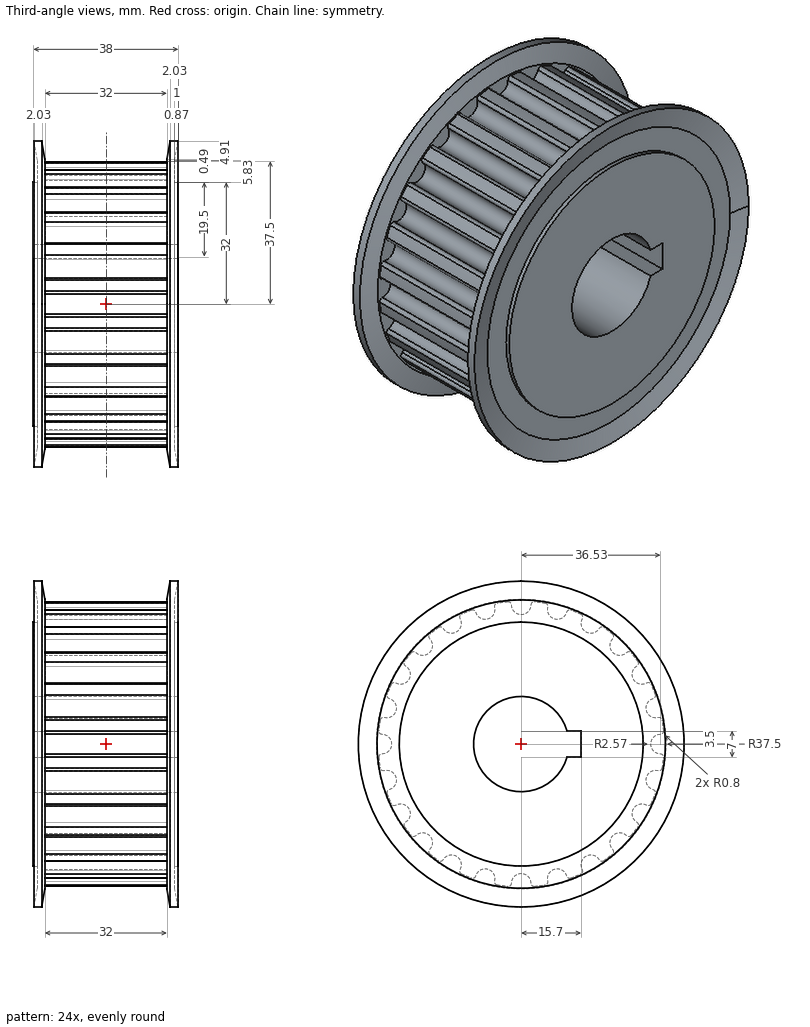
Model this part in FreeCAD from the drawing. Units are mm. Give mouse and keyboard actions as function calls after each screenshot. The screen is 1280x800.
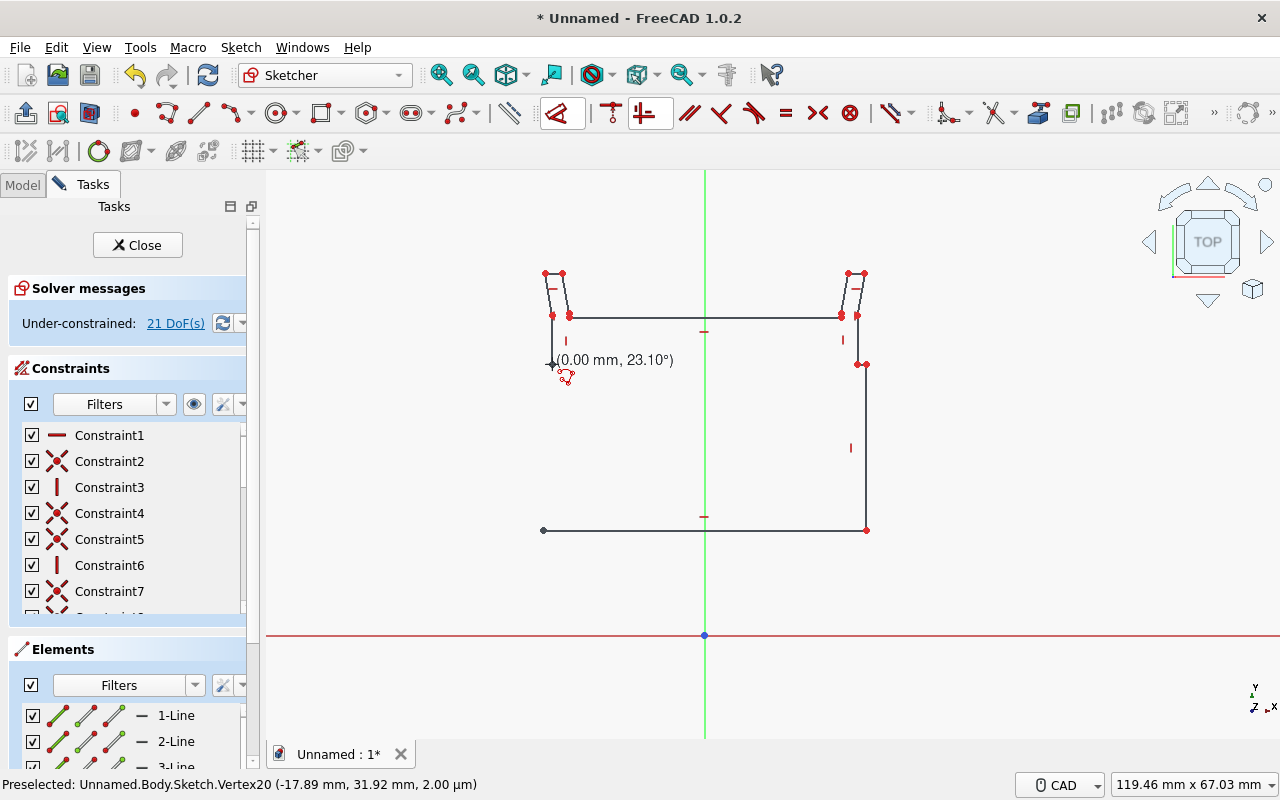
scroll(544, 364, up, 4)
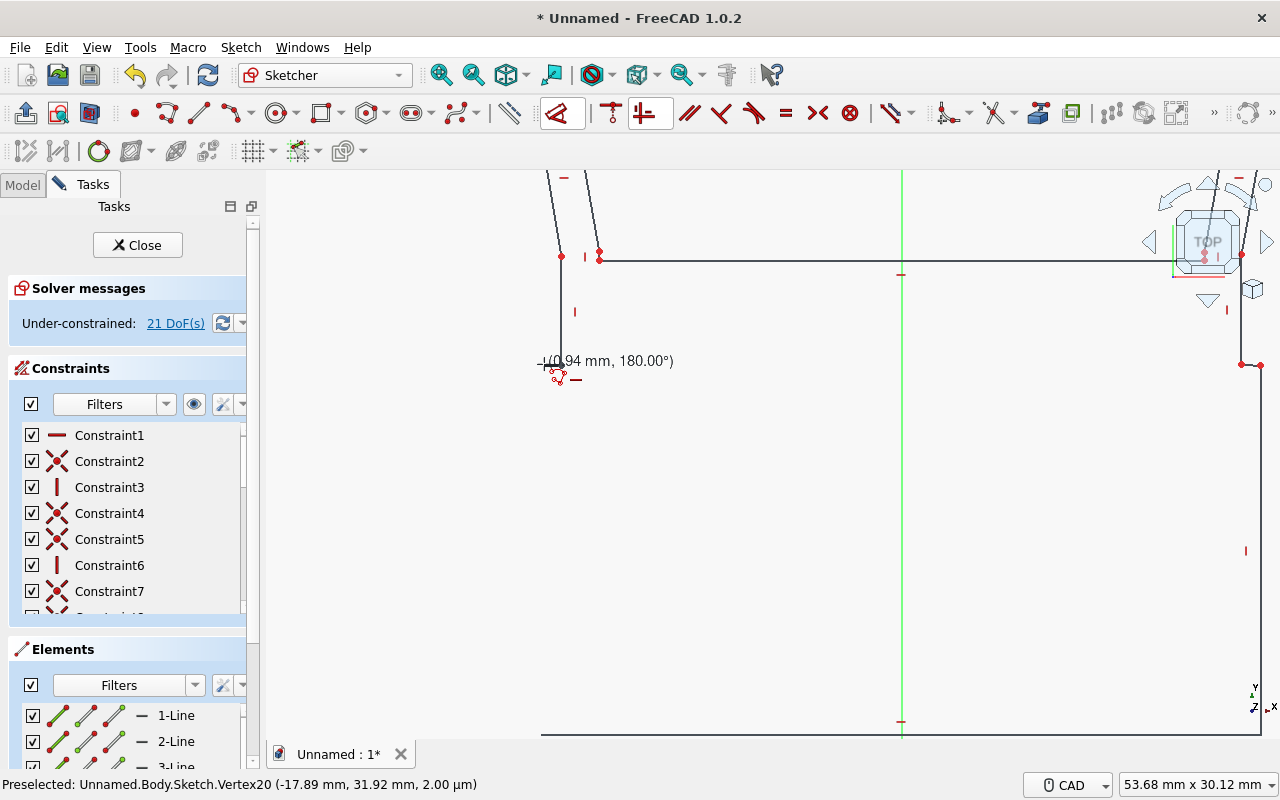
click(543, 364)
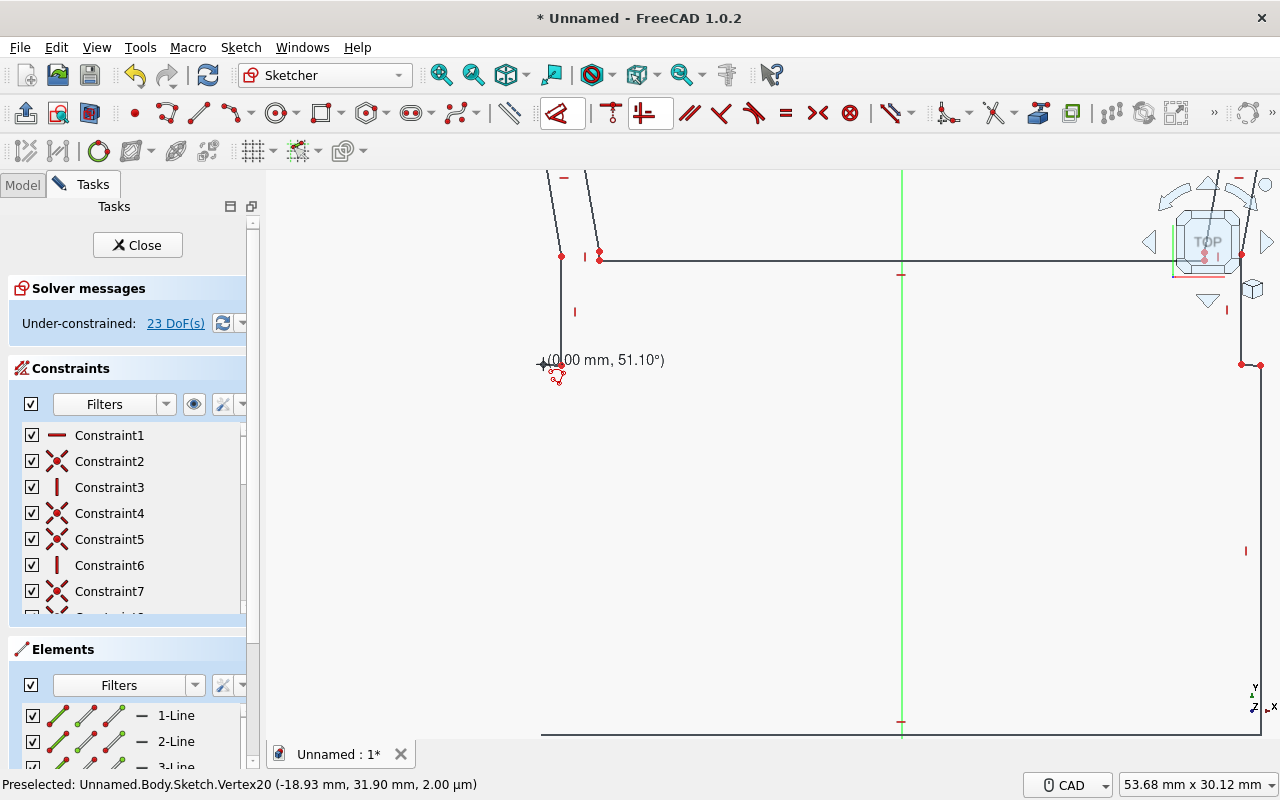
scroll(544, 364, down, 4)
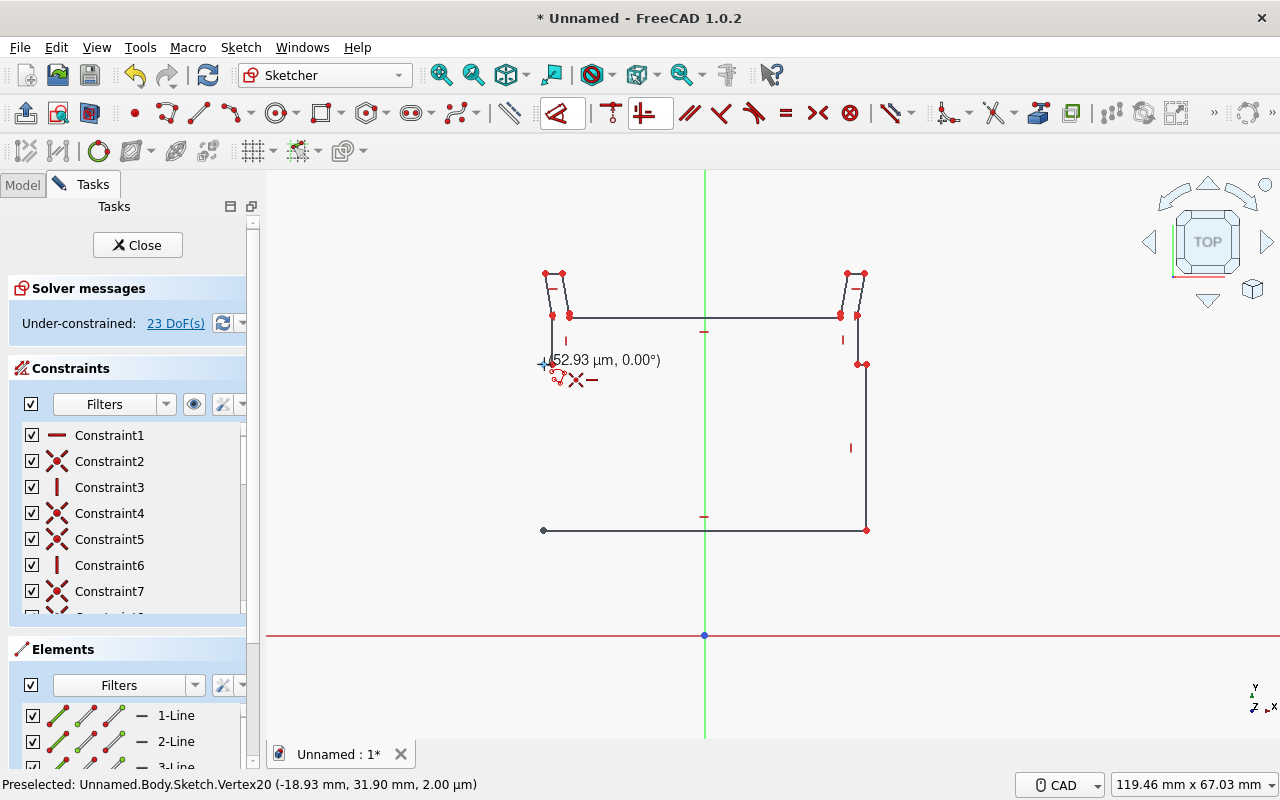
click(543, 531)
key(Escape)
key(Escape)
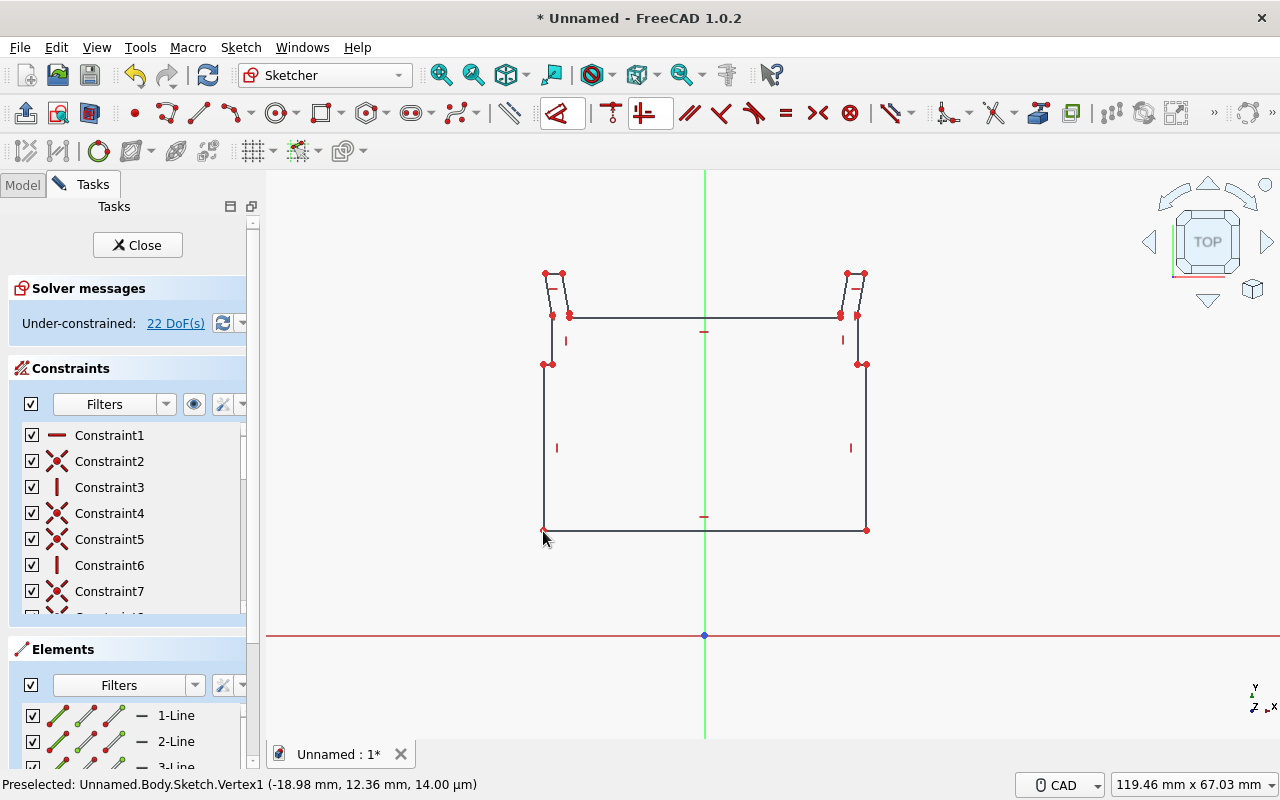
scroll(862, 365, up, 6)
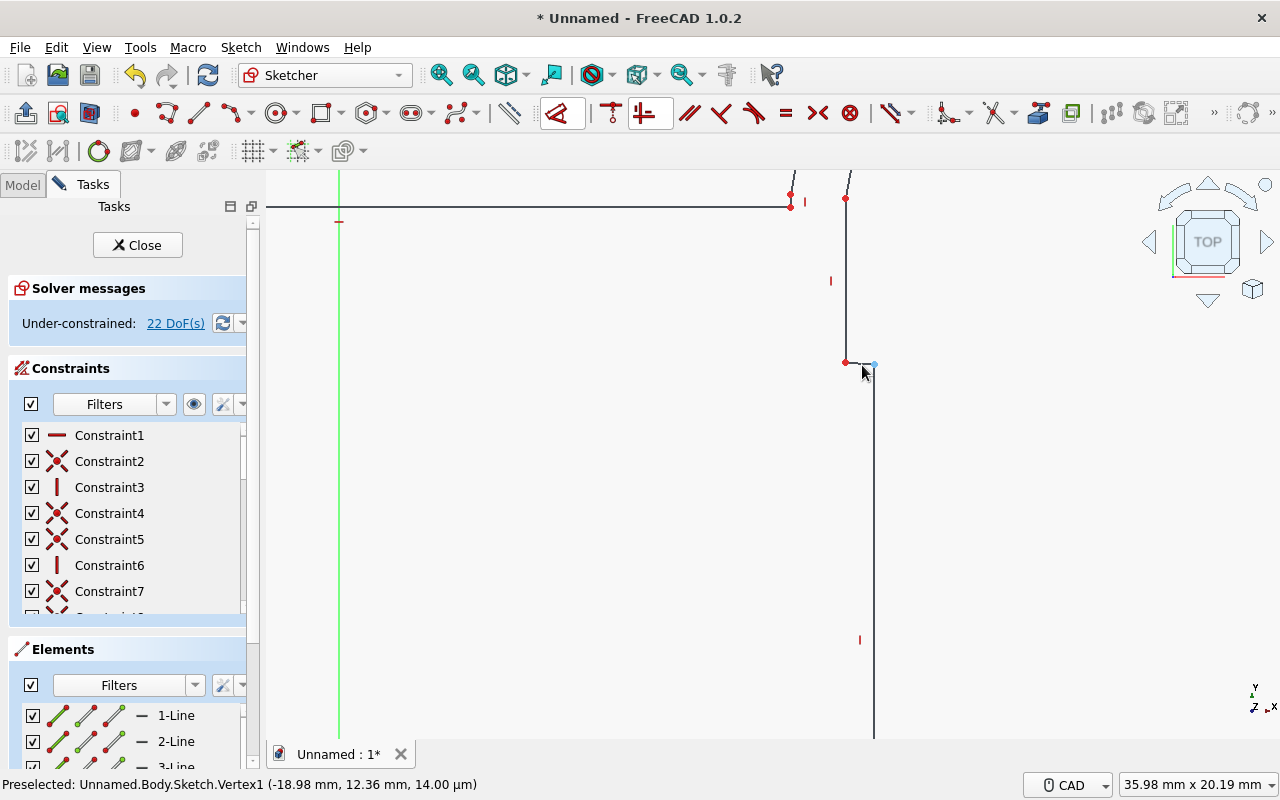
click(860, 364)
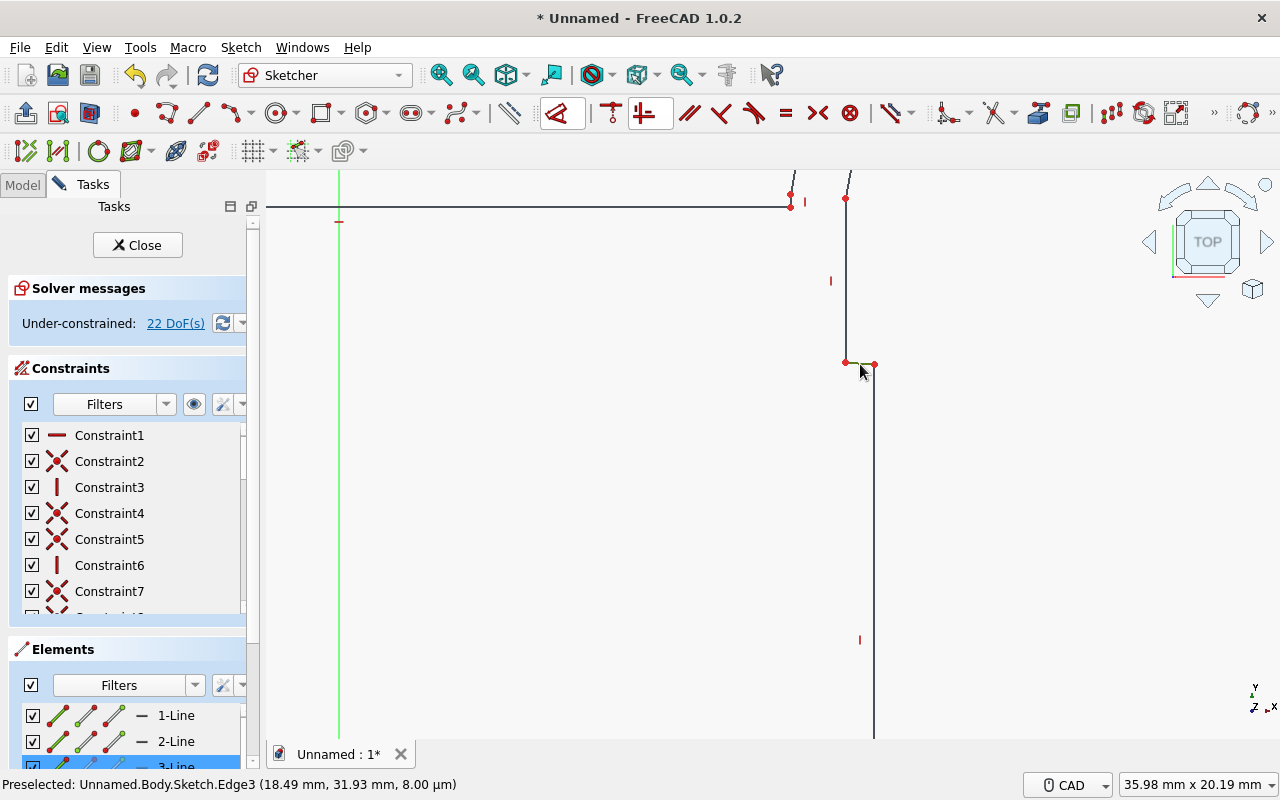
click(668, 114)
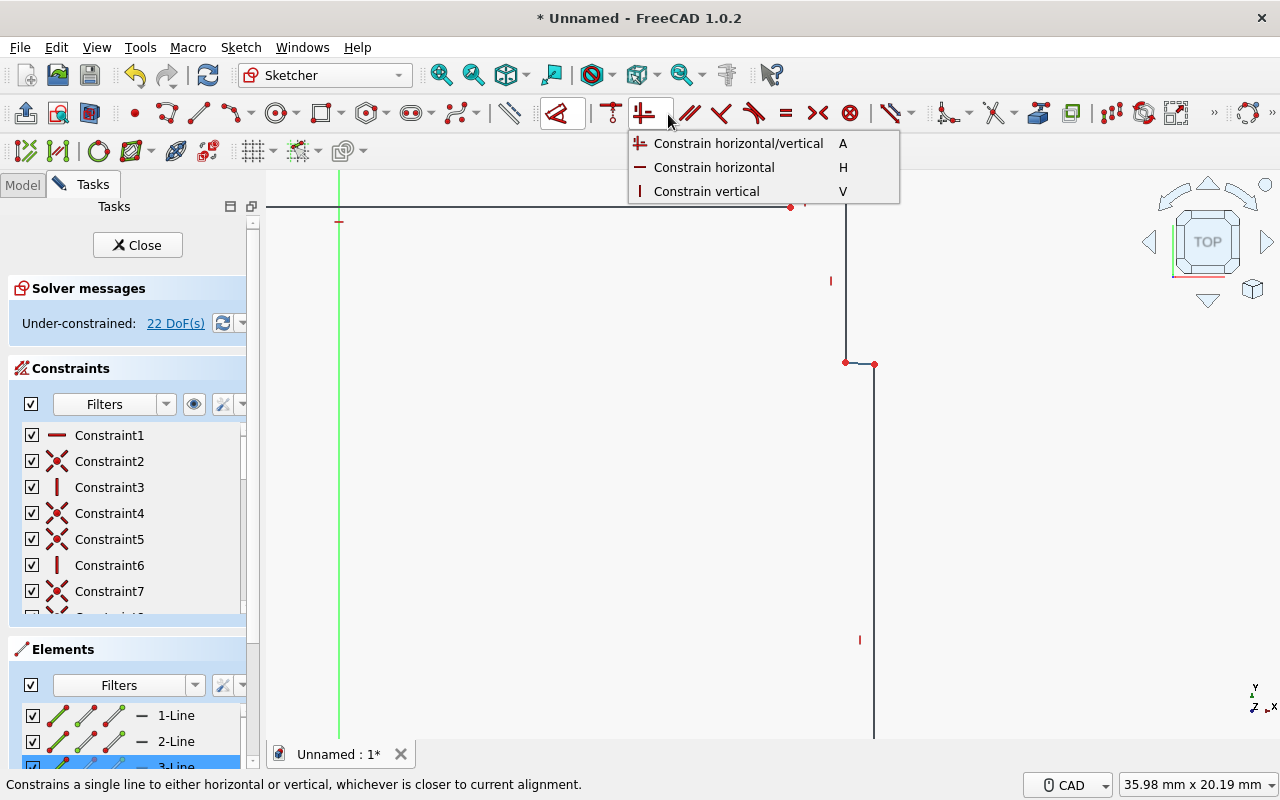
click(764, 167)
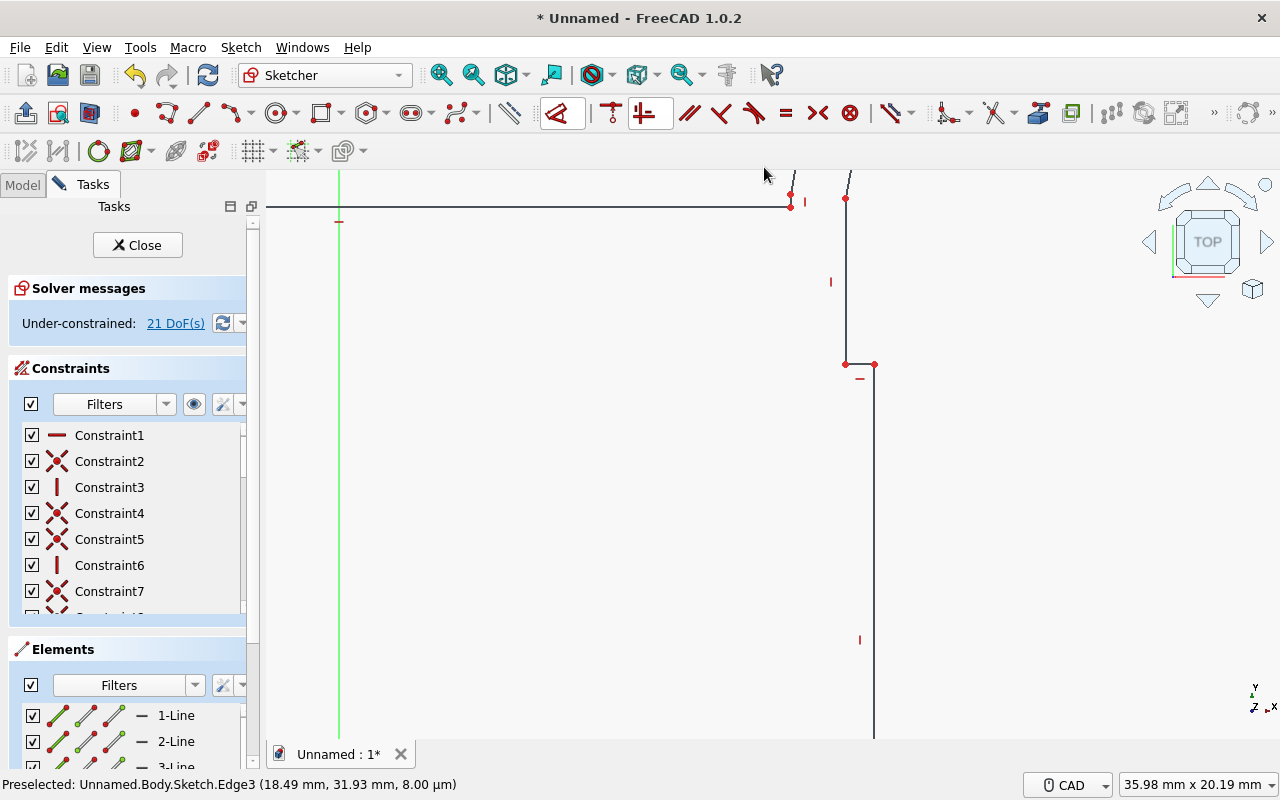
scroll(862, 365, down, 6)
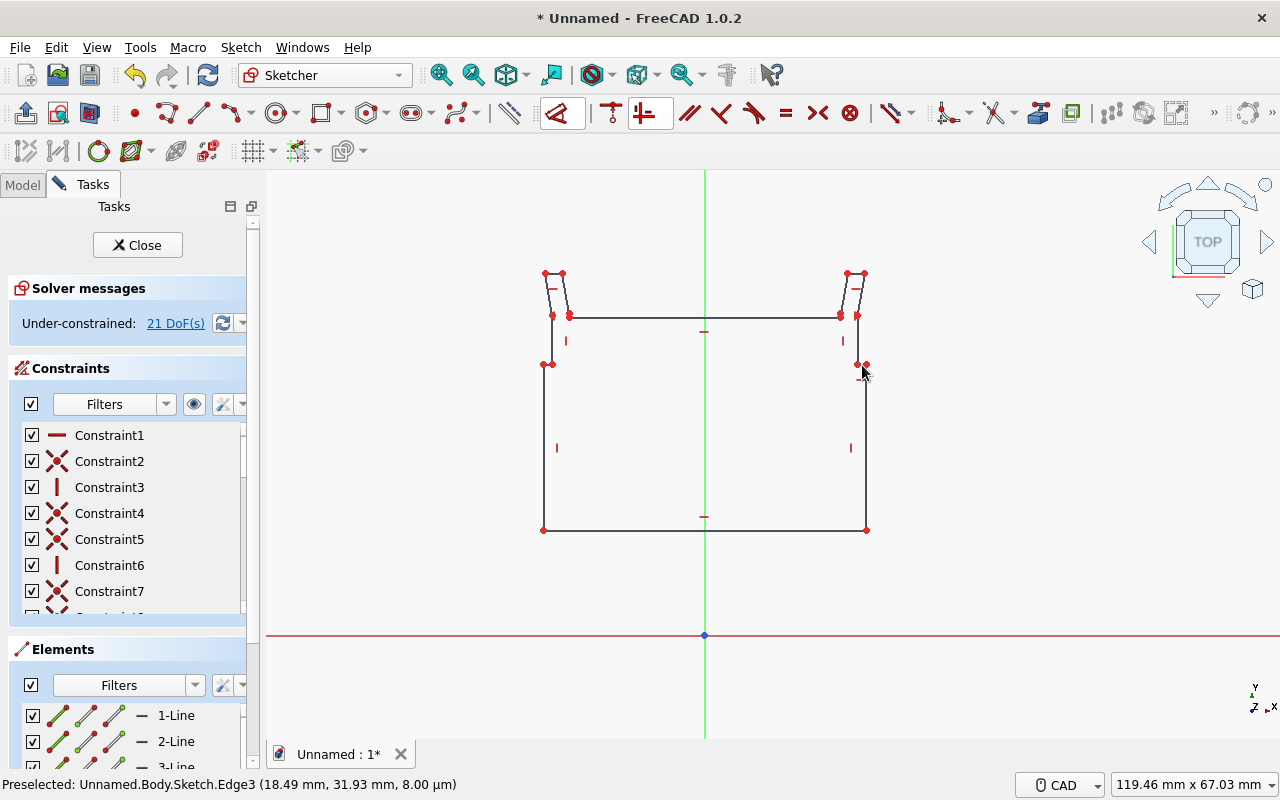
scroll(549, 365, up, 8)